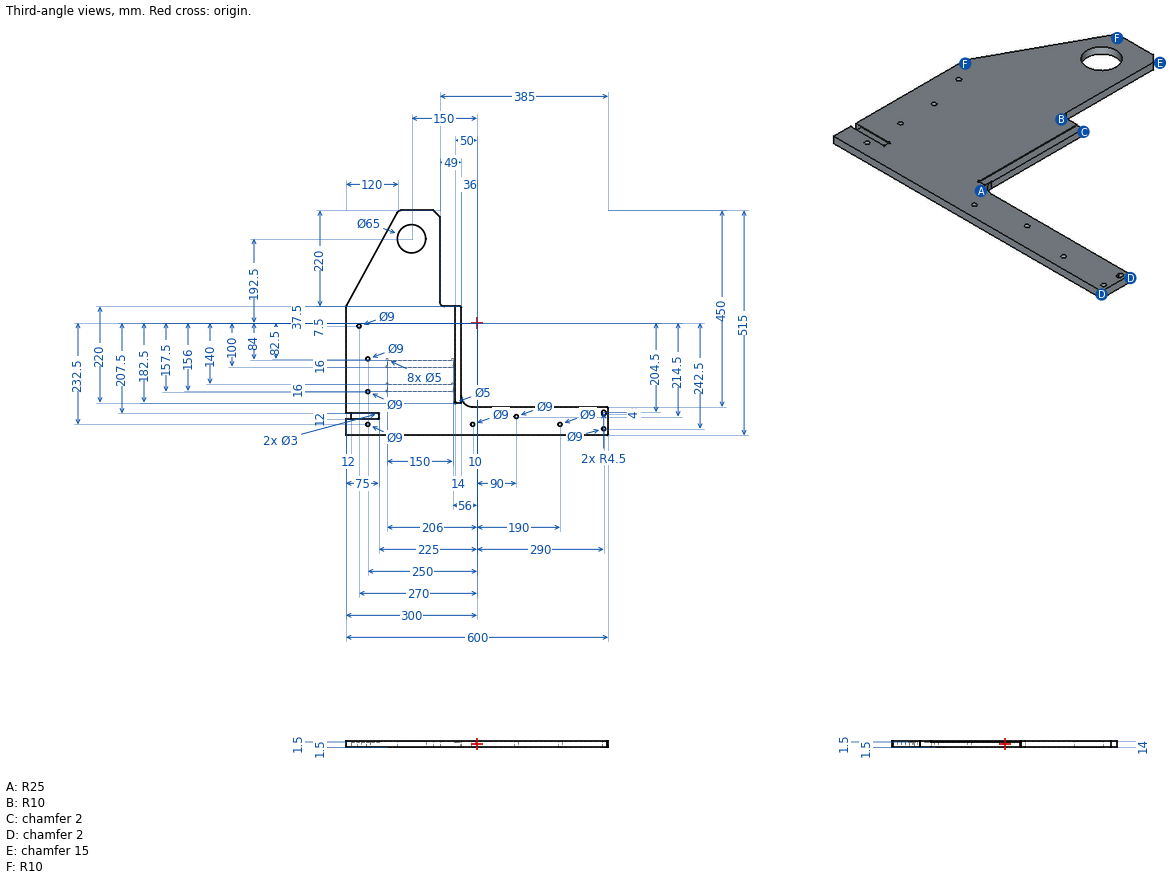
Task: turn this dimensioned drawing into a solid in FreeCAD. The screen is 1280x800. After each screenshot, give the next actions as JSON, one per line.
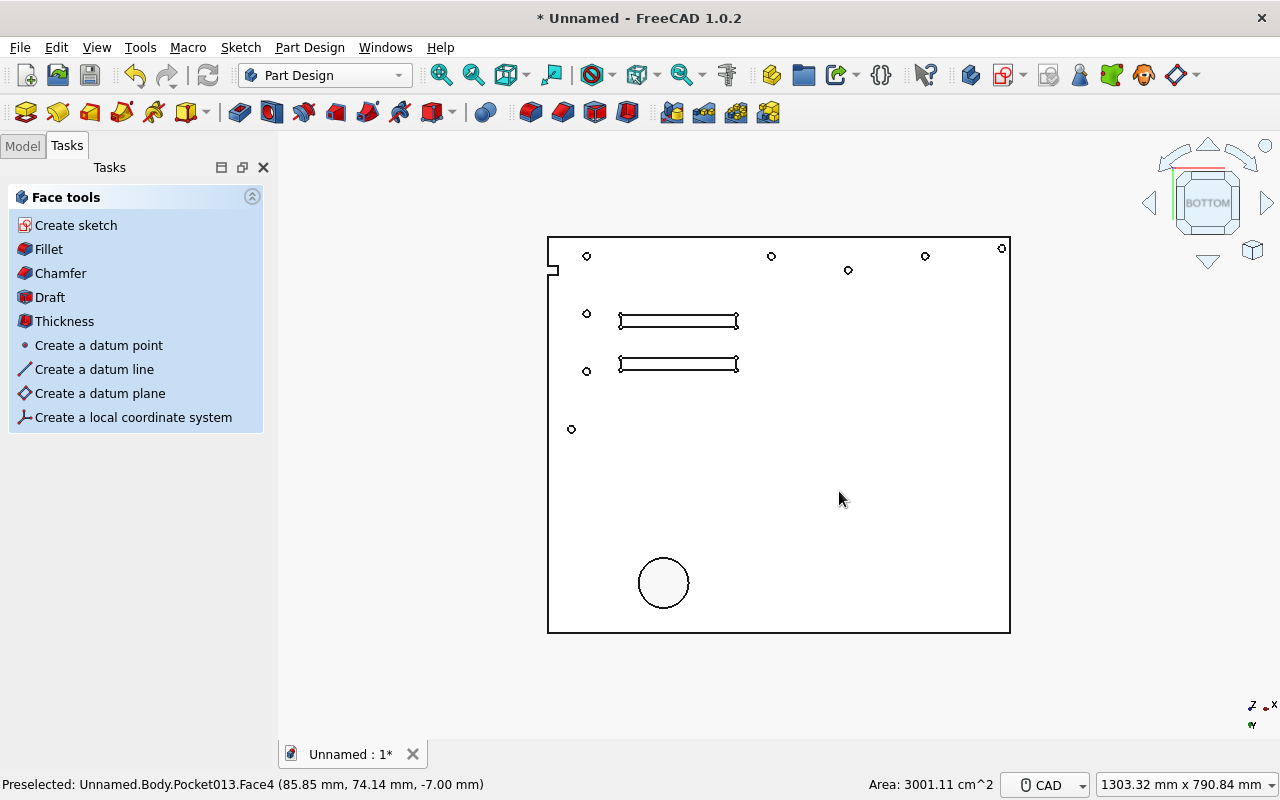
{"action": "left_click", "coordinate": [1004, 76]}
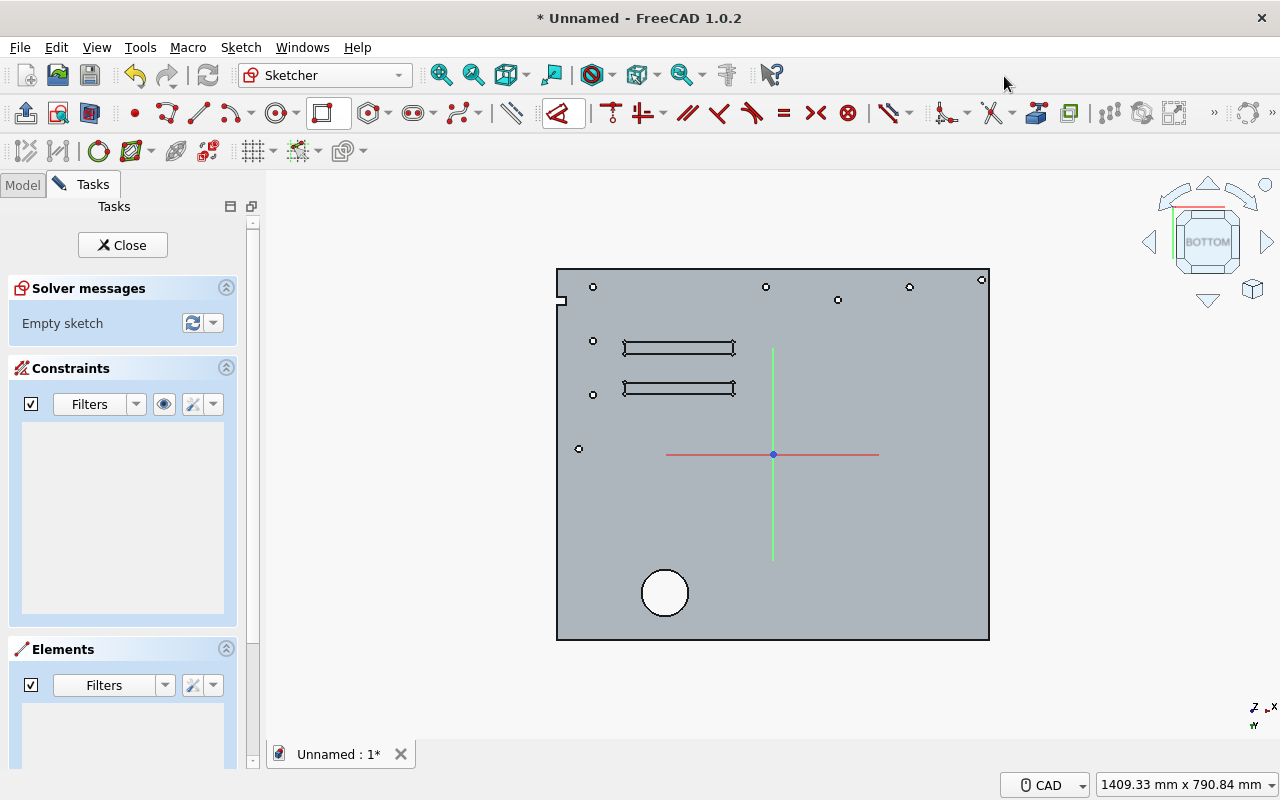
{"action": "scroll", "coordinate": [996, 298], "scroll_direction": "up", "scroll_amount": 15}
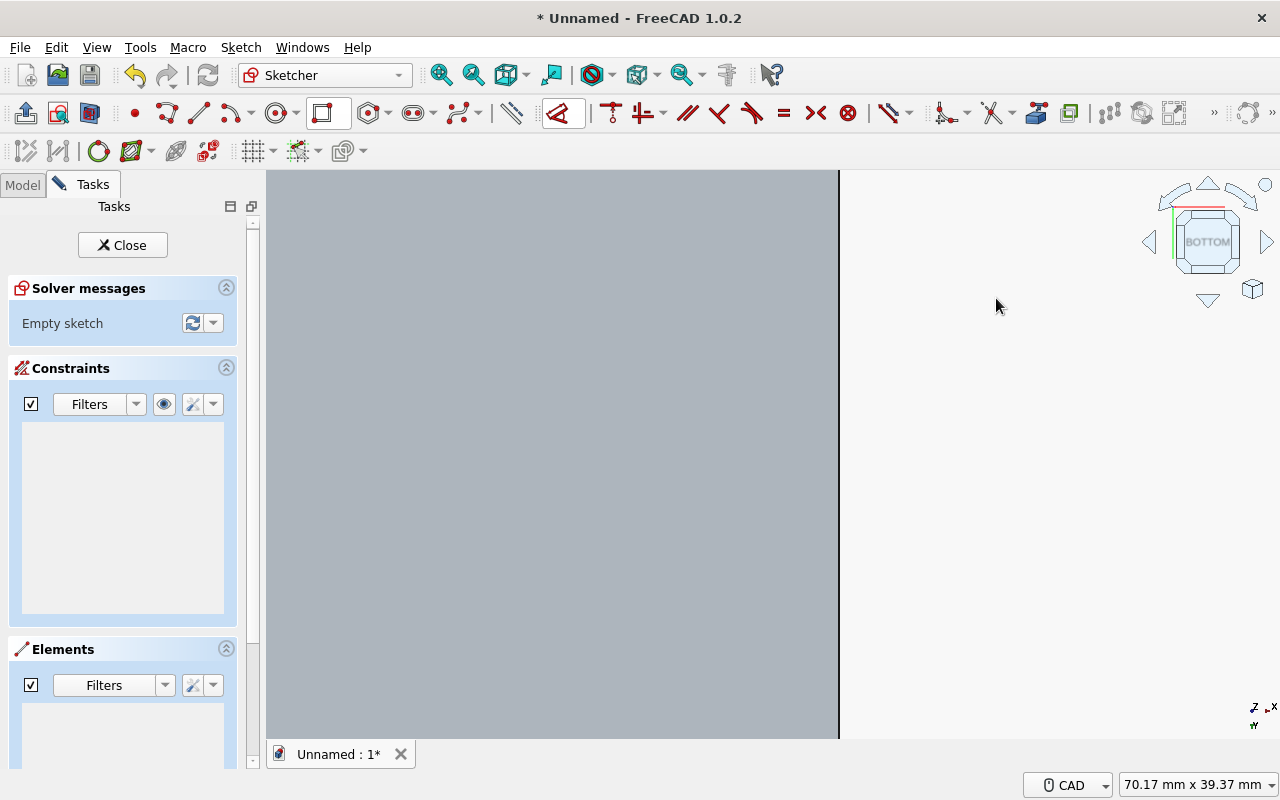
{"action": "scroll", "coordinate": [681, 451], "scroll_direction": "up", "scroll_amount": 3}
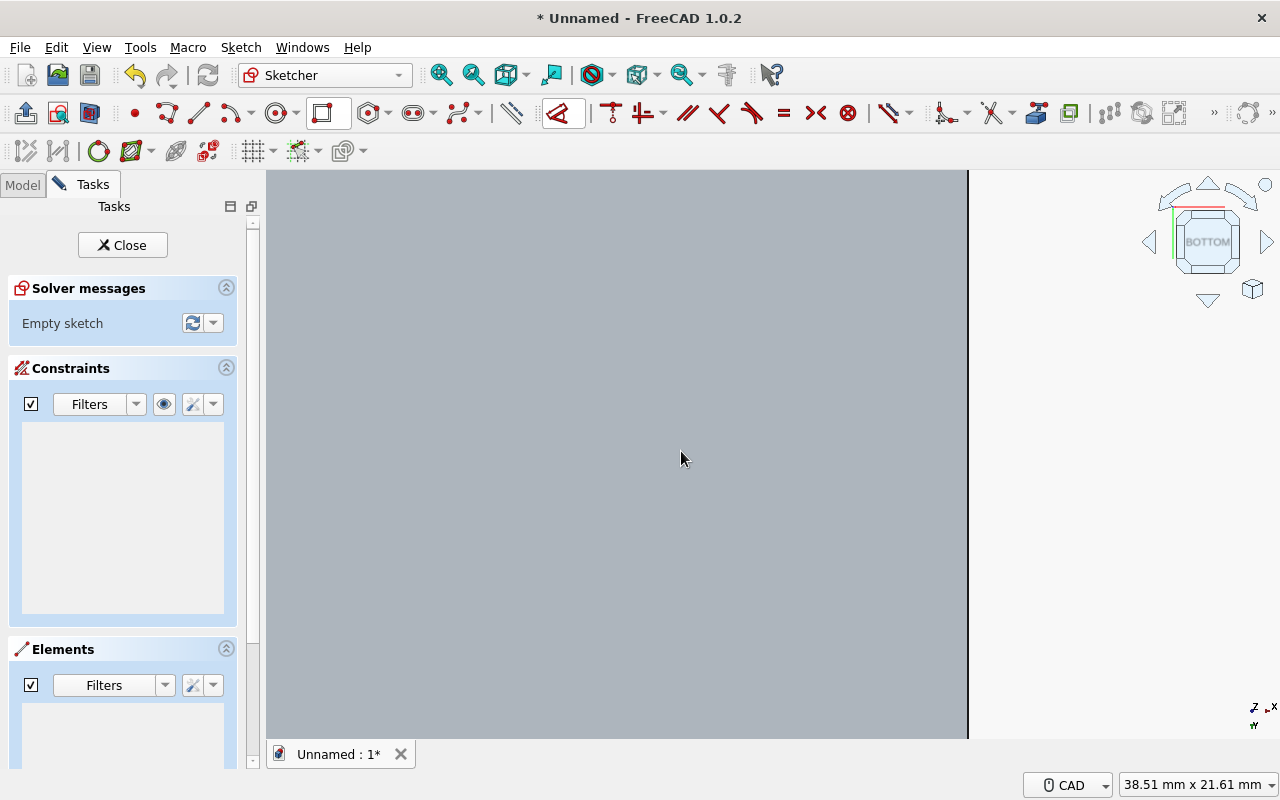
{"action": "left_click", "coordinate": [414, 114]}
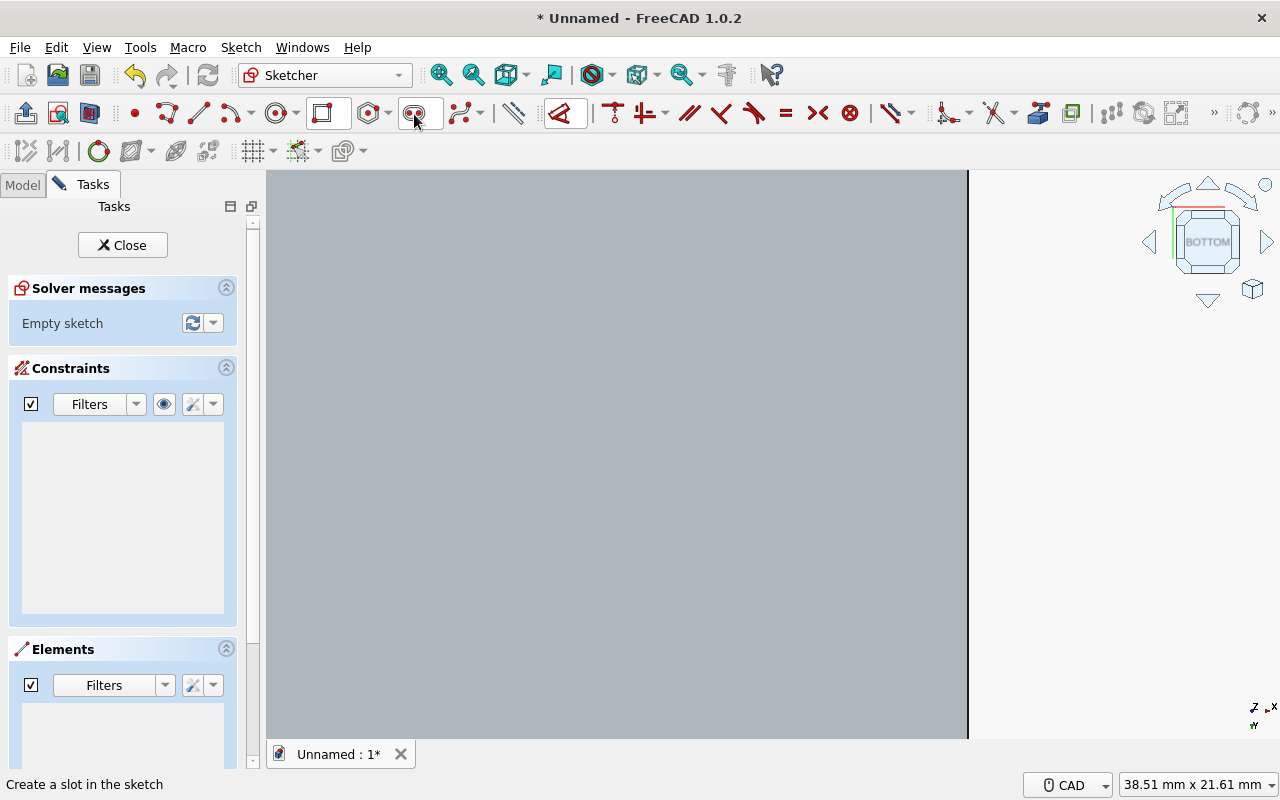
{"action": "left_click", "coordinate": [704, 507]}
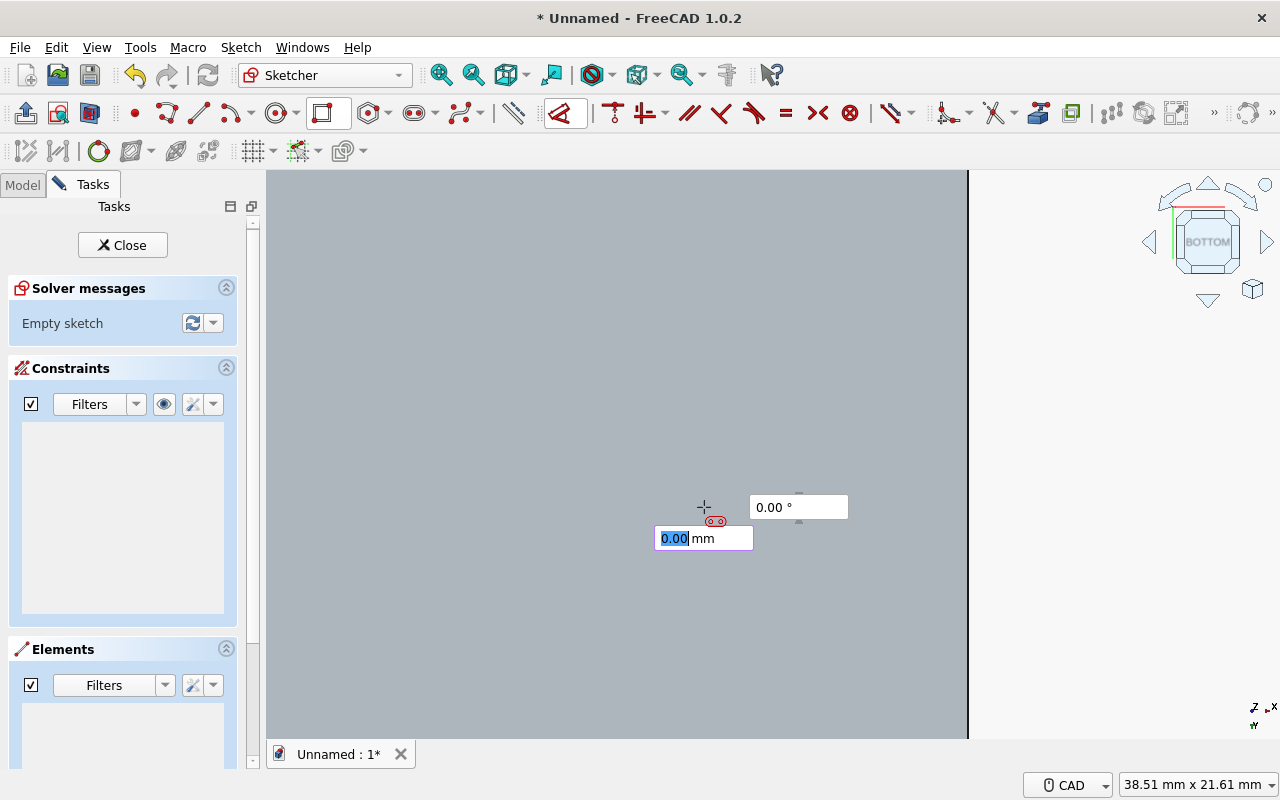
{"action": "left_click", "coordinate": [704, 401]}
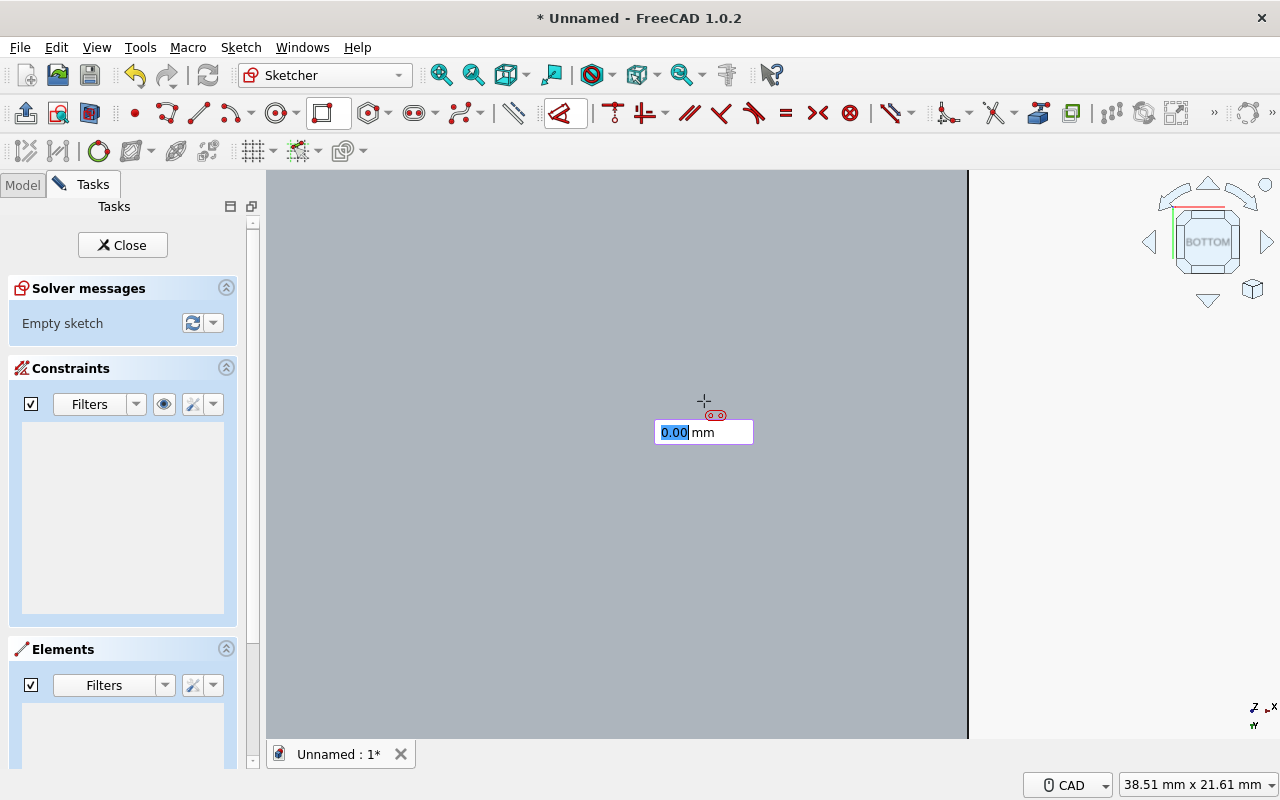
{"action": "left_click", "coordinate": [586, 454]}
{"action": "key", "text": "Escape"}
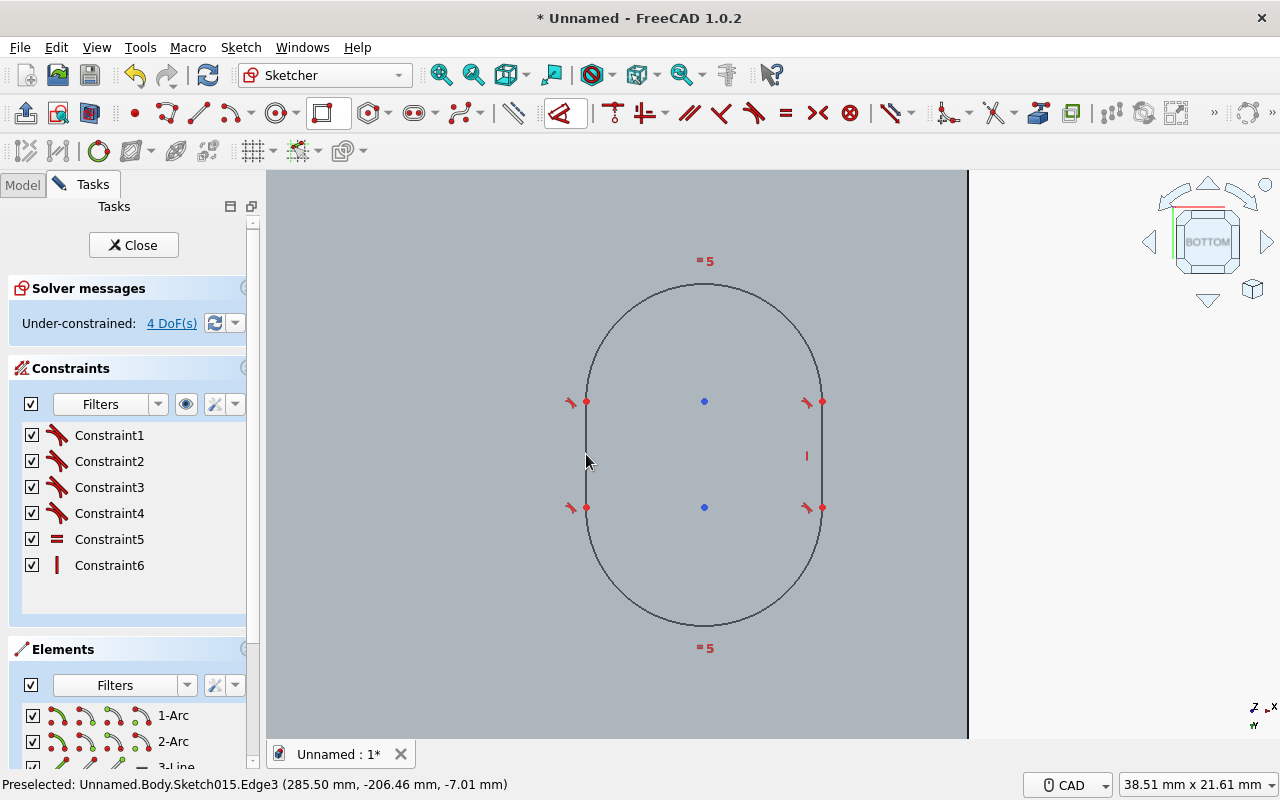
{"action": "left_click", "coordinate": [635, 603]}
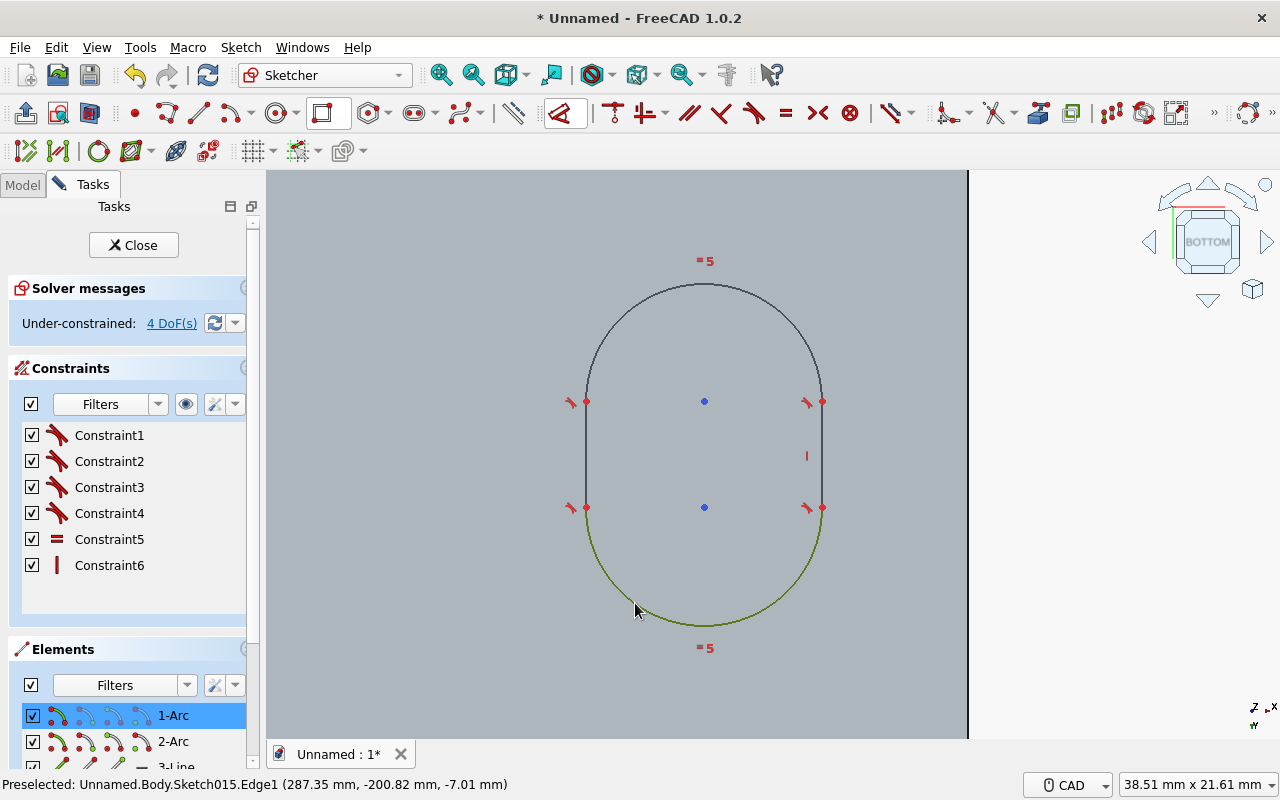
{"action": "left_click", "coordinate": [582, 114]}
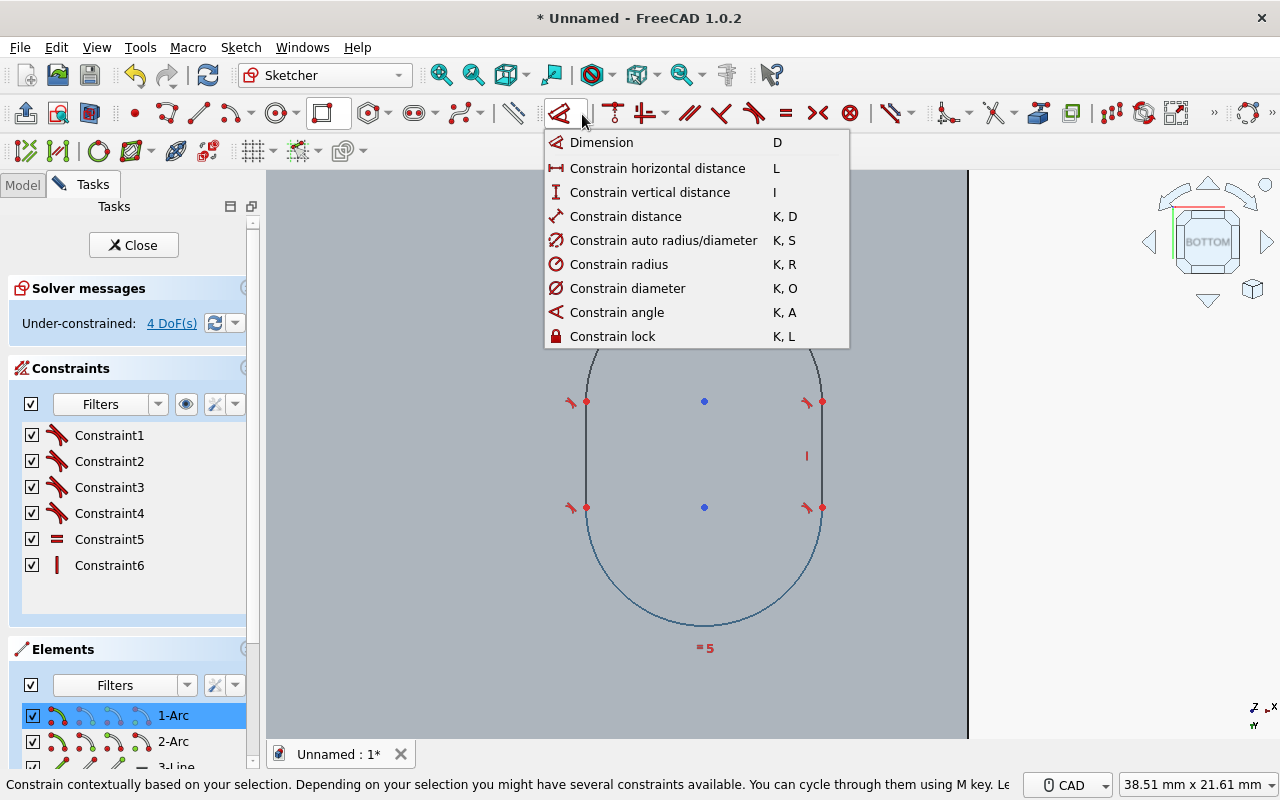
{"action": "left_click", "coordinate": [697, 264]}